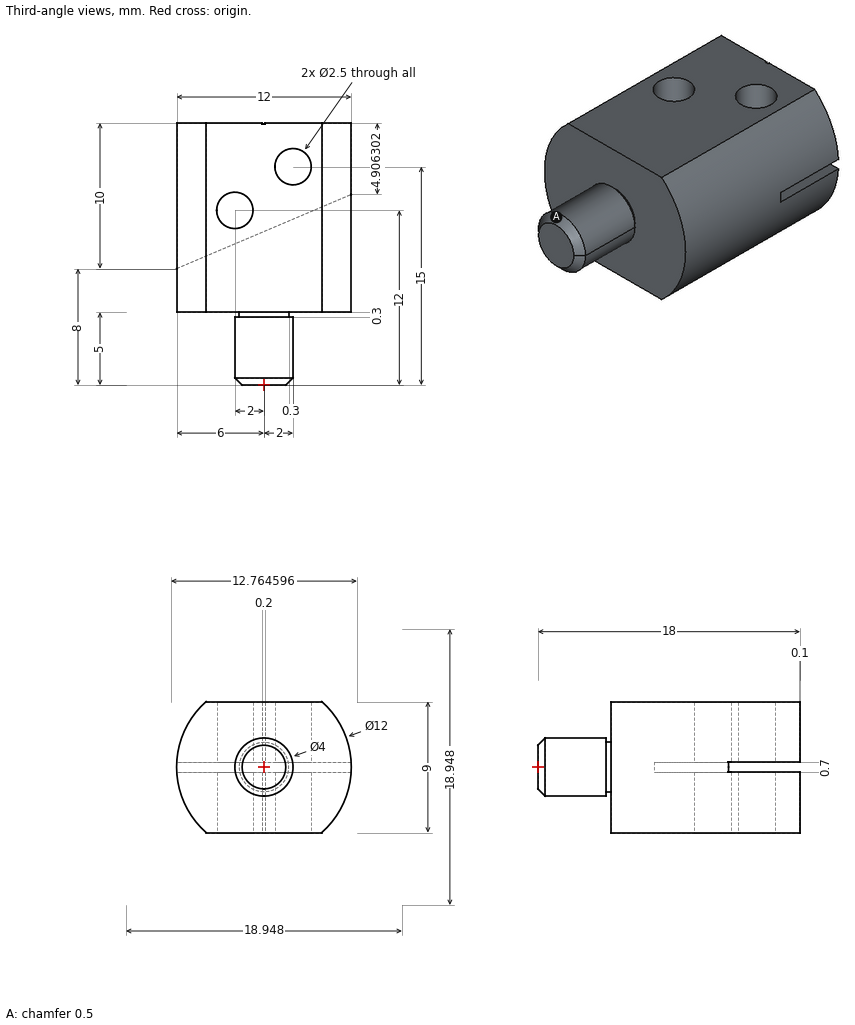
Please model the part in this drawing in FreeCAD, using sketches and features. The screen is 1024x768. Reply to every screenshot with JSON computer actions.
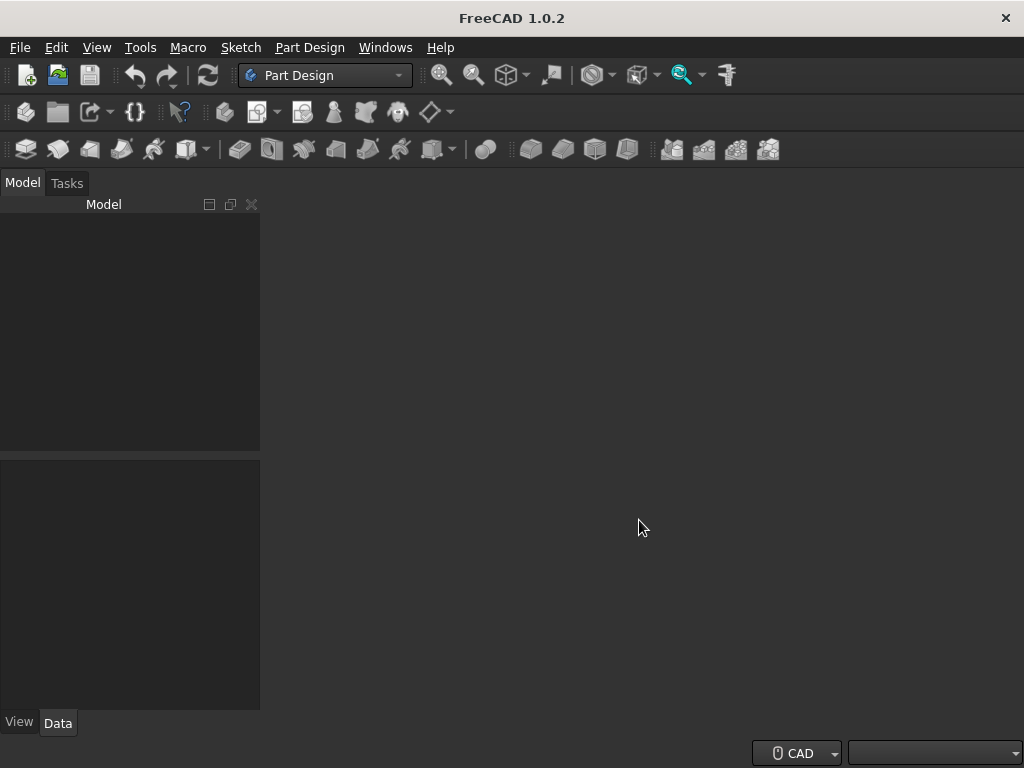
{"action": "key", "text": "ctrl+n"}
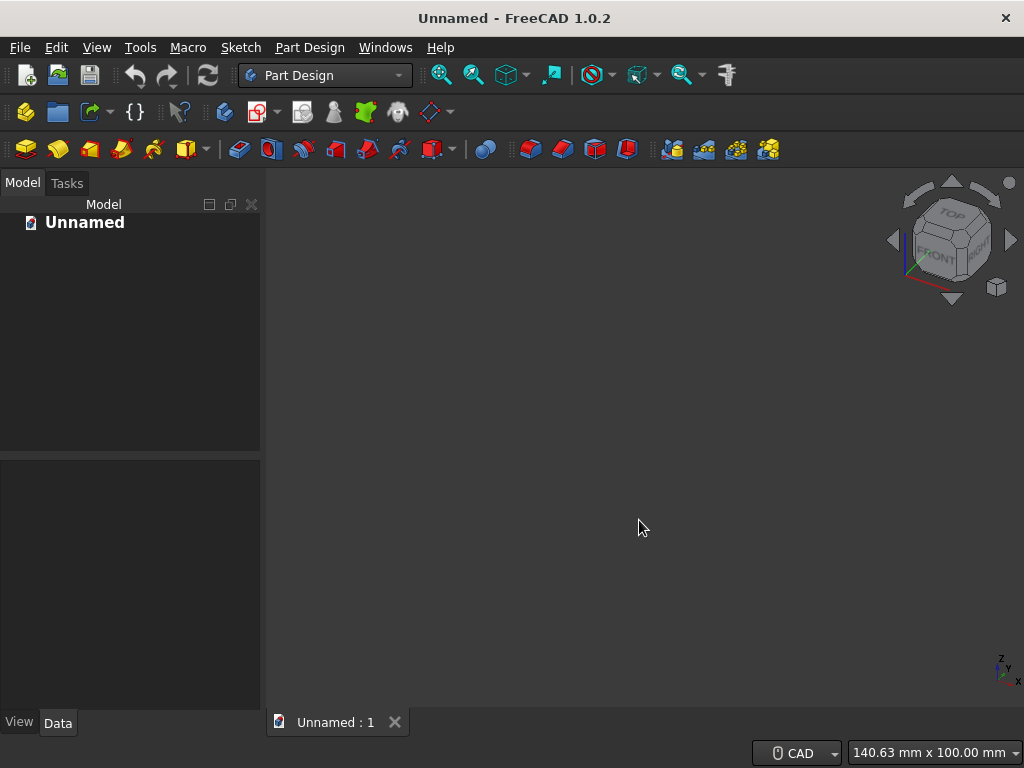
{"action": "left_click", "coordinate": [258, 112]}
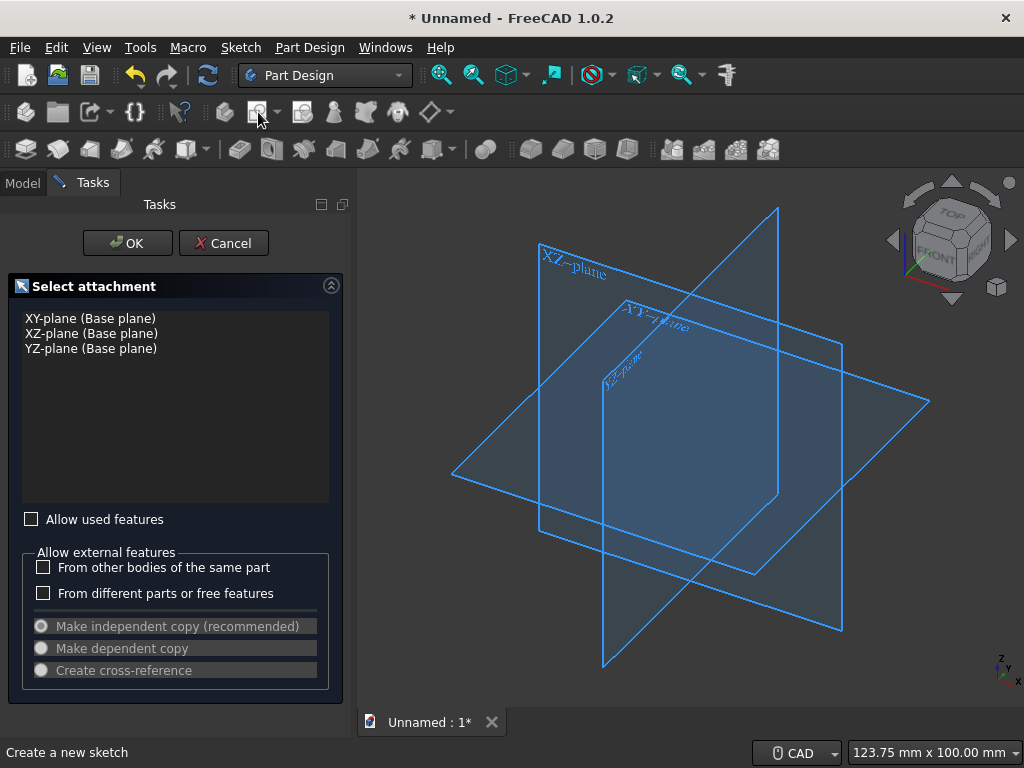
{"action": "left_click", "coordinate": [82, 334]}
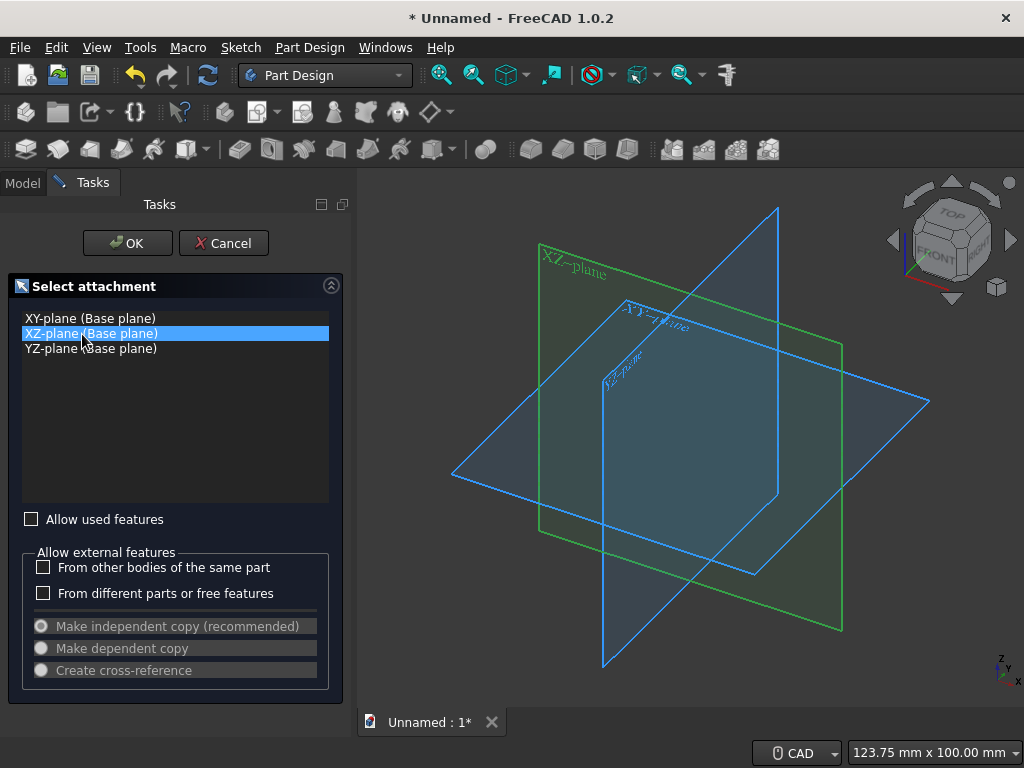
{"action": "left_click", "coordinate": [128, 243]}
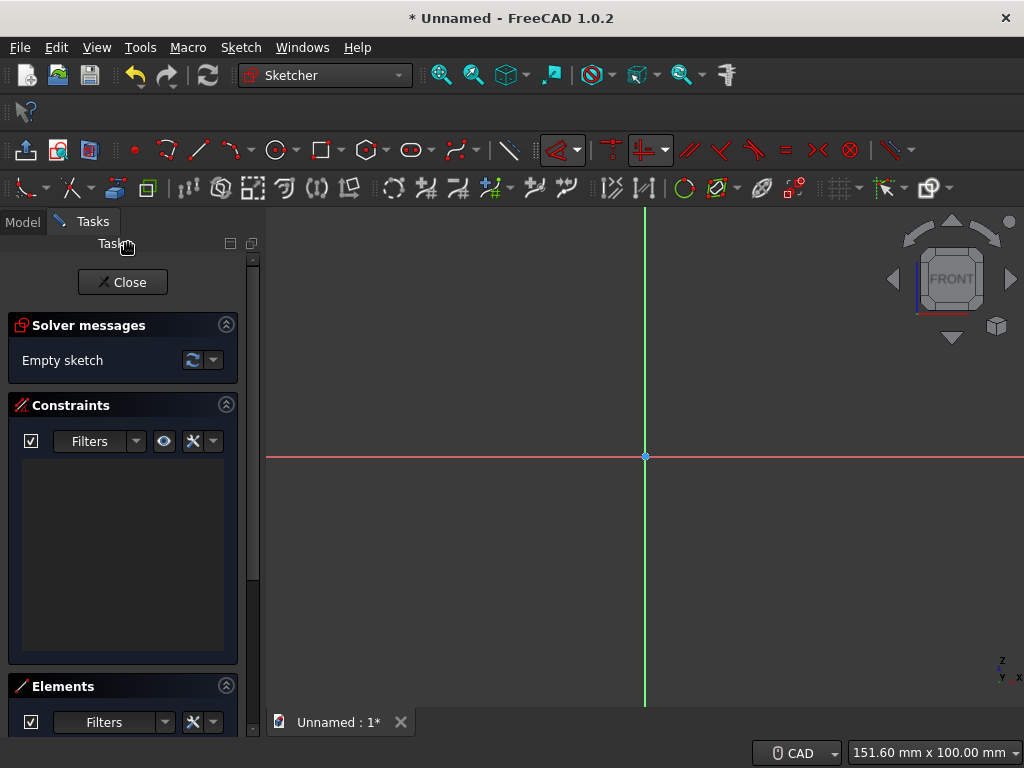
{"action": "scroll", "coordinate": [662, 457], "scroll_direction": "up", "scroll_amount": 8}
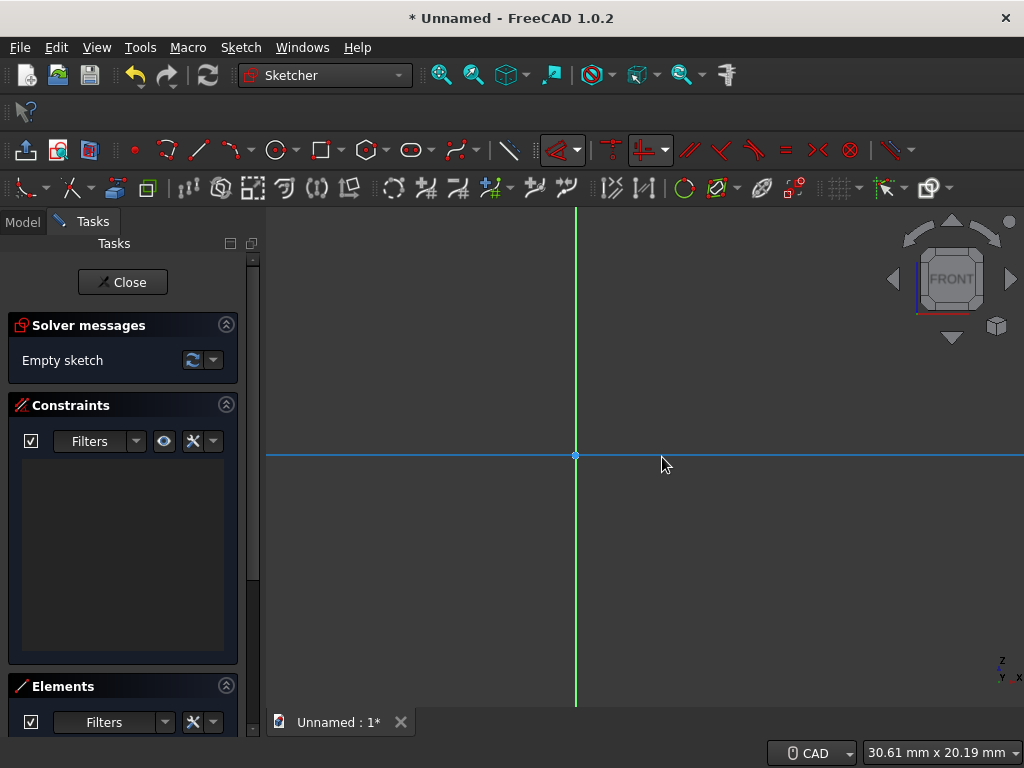
{"action": "key", "text": "g c"}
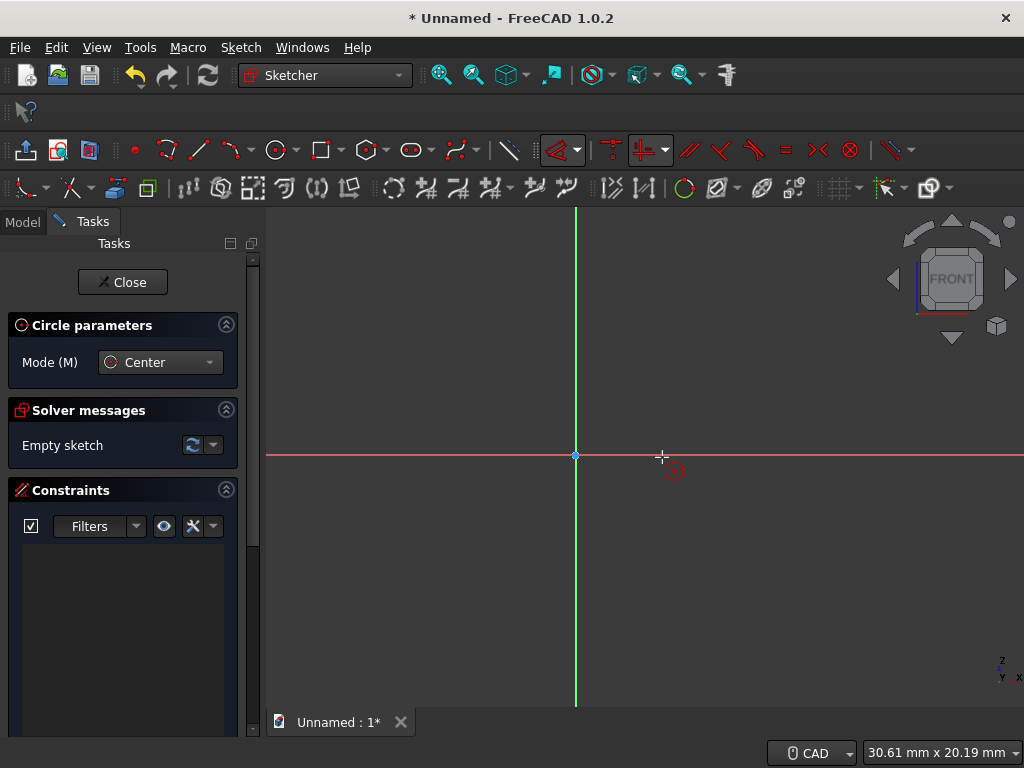
{"action": "left_click", "coordinate": [576, 455]}
{"action": "left_click", "coordinate": [681, 350]}
{"action": "key", "text": "Escape"}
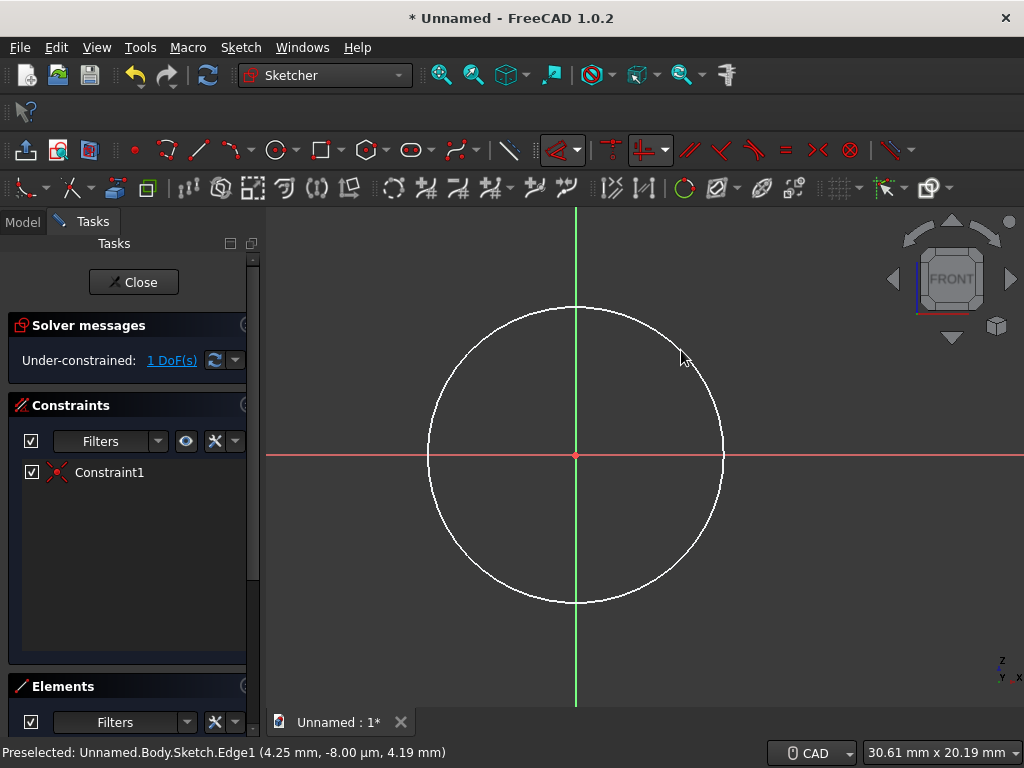
{"action": "left_click", "coordinate": [680, 350]}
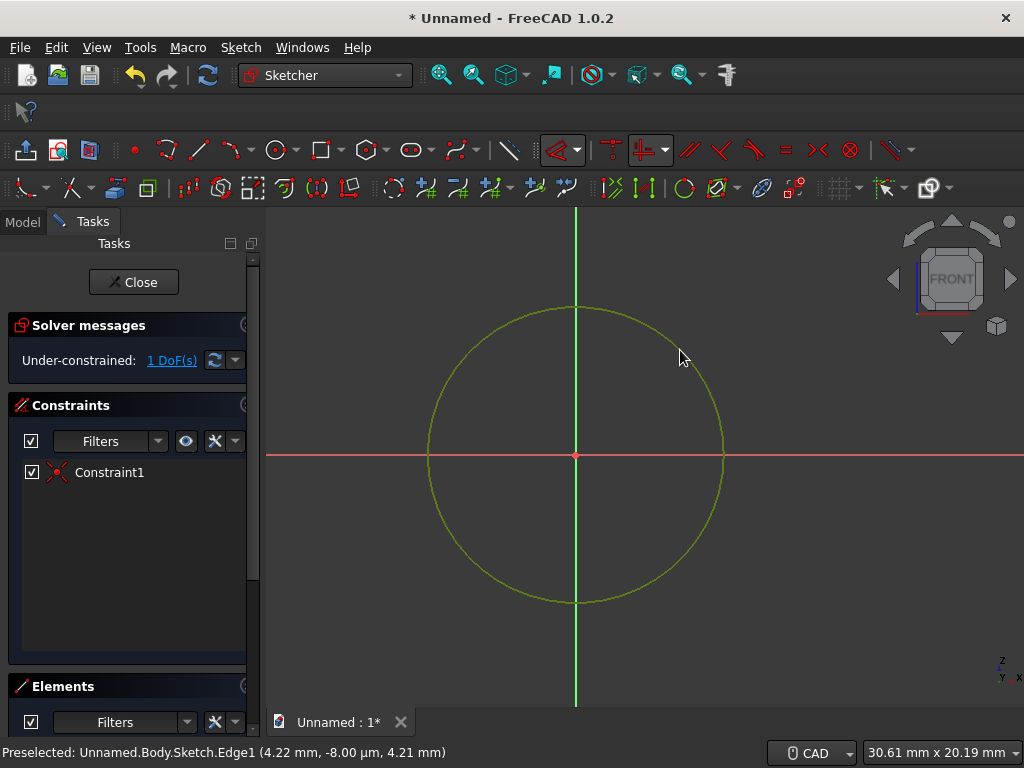
{"action": "left_click", "coordinate": [580, 150]}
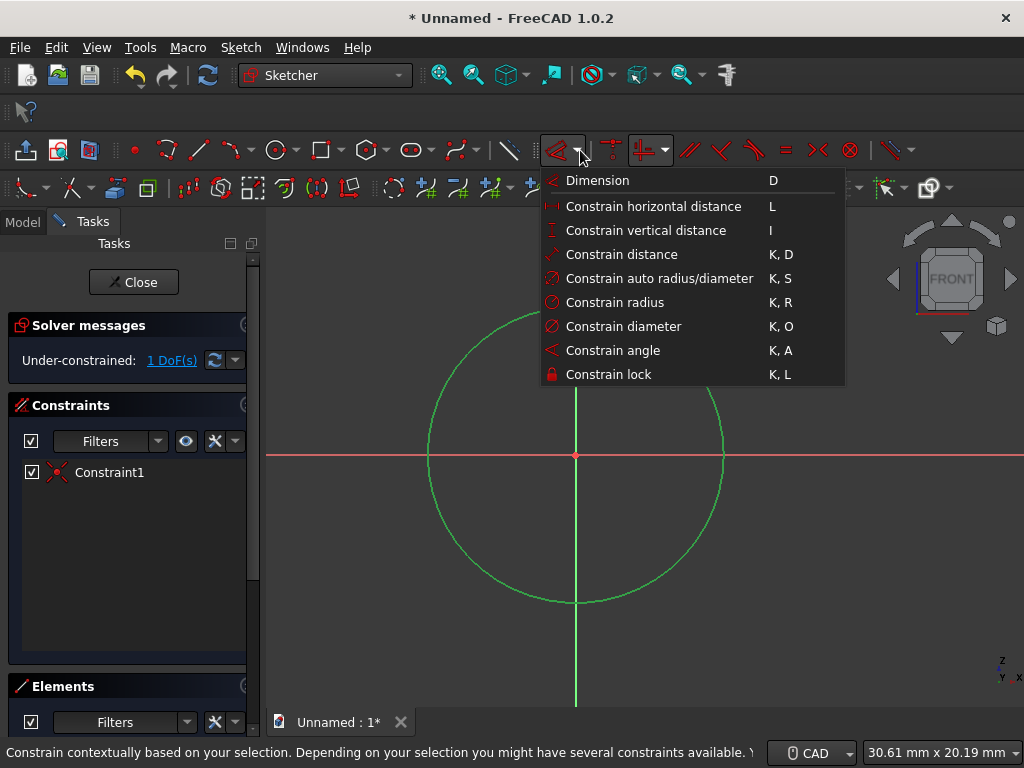
{"action": "left_click", "coordinate": [693, 326]}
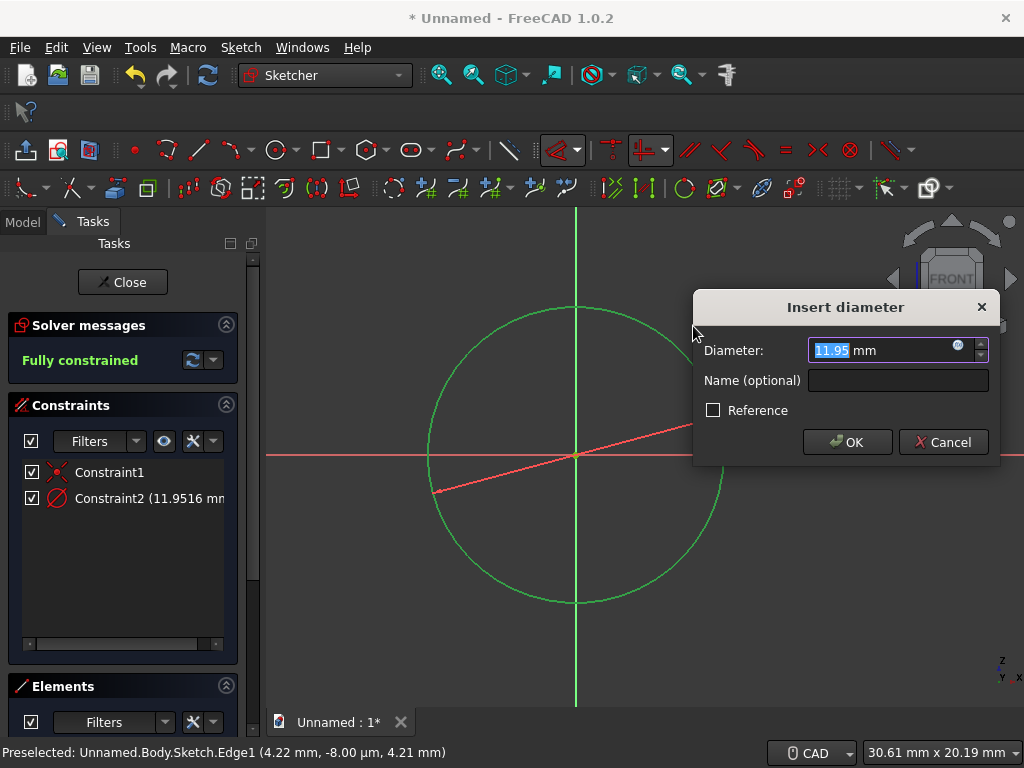
{"action": "type", "text": "12"}
{"action": "key", "text": "Return"}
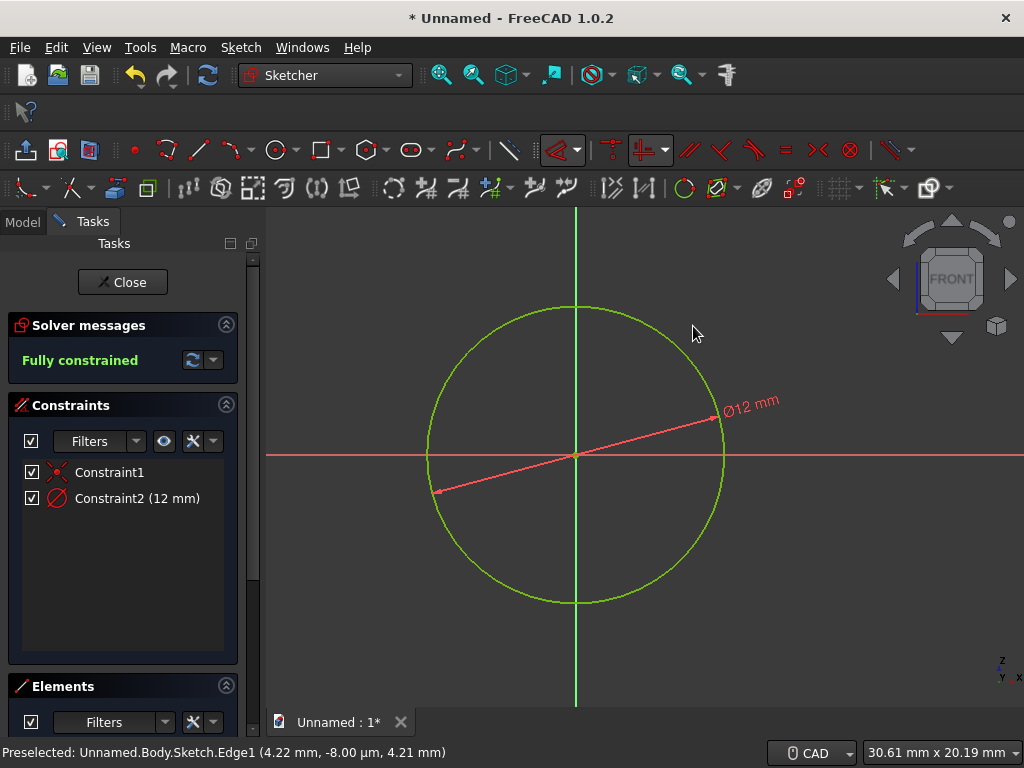
{"action": "left_click", "coordinate": [123, 282]}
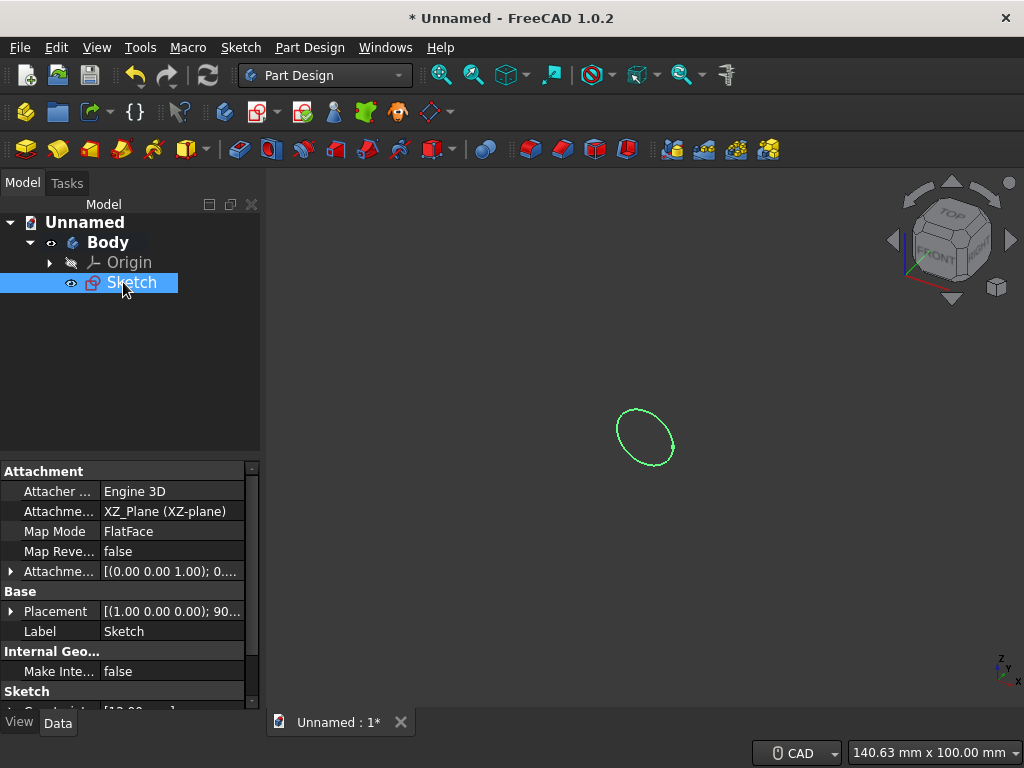
{"action": "left_click", "coordinate": [26, 150]}